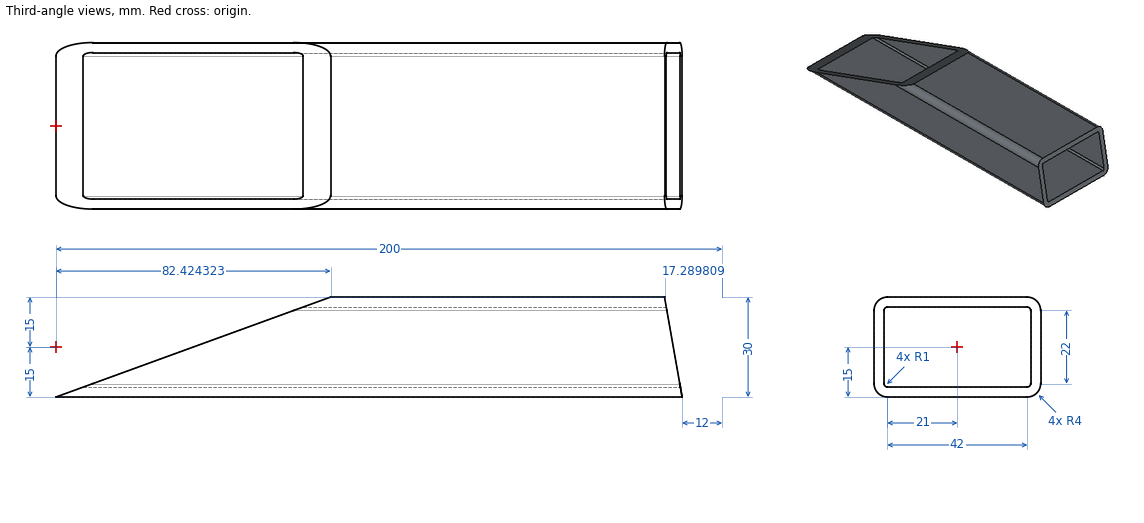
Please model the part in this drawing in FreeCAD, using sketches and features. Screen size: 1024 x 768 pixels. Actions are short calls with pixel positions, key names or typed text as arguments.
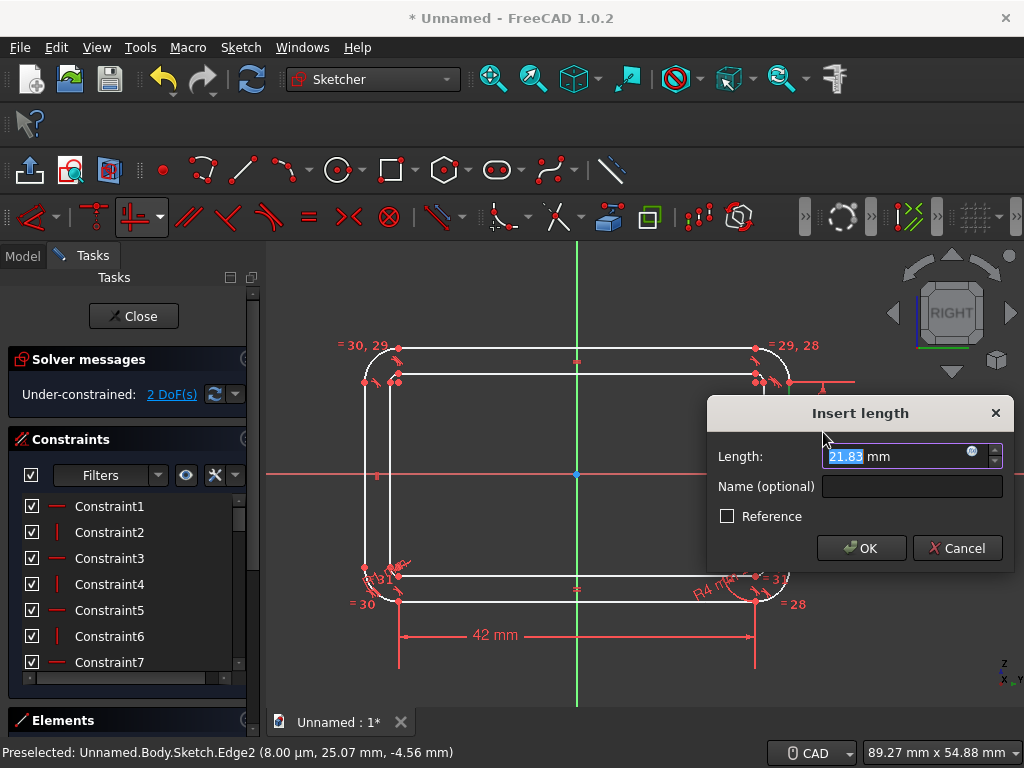
text(22)
key(Return)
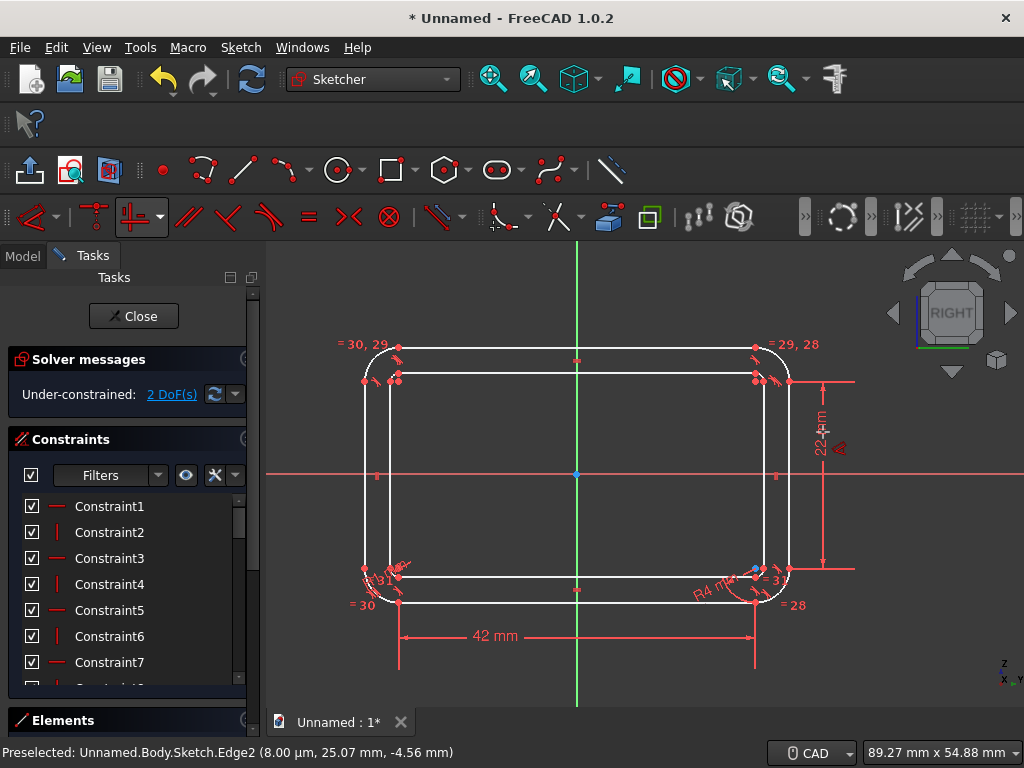
click(399, 603)
click(426, 637)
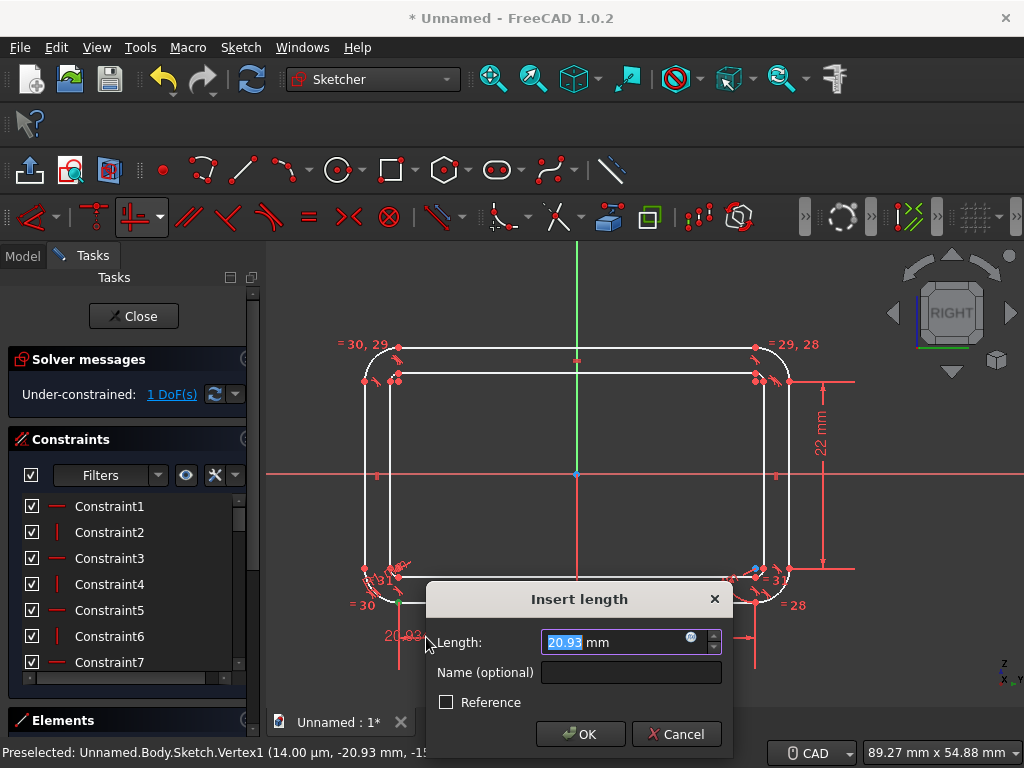
text(21)
key(Return)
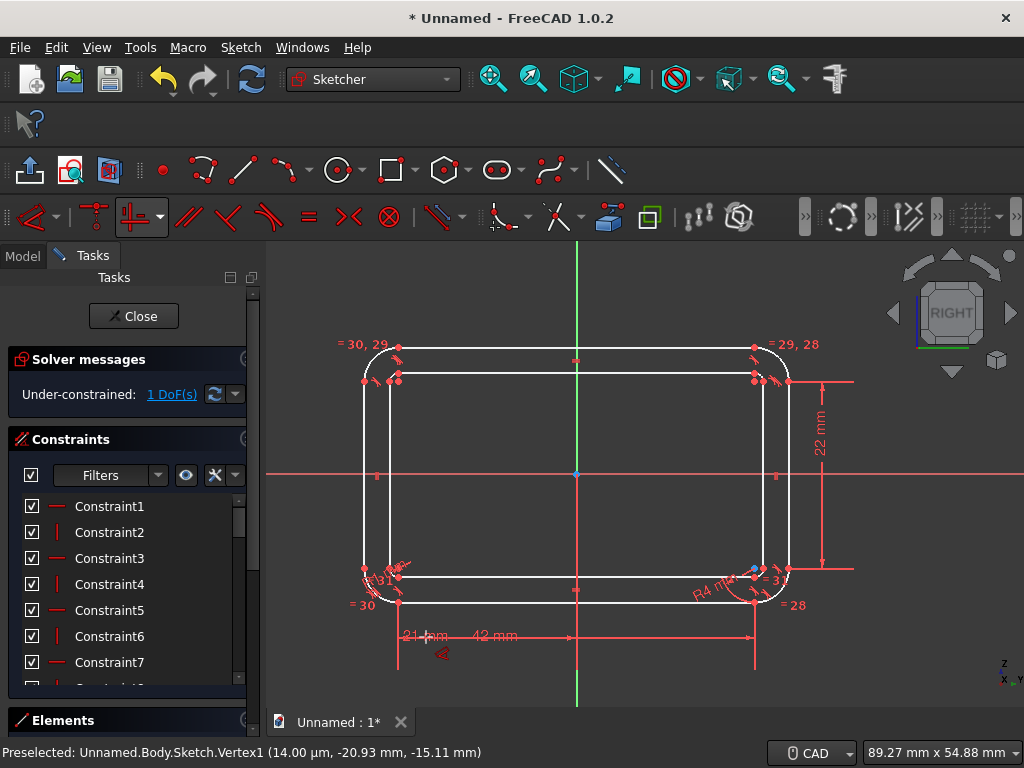
click(398, 603)
click(611, 538)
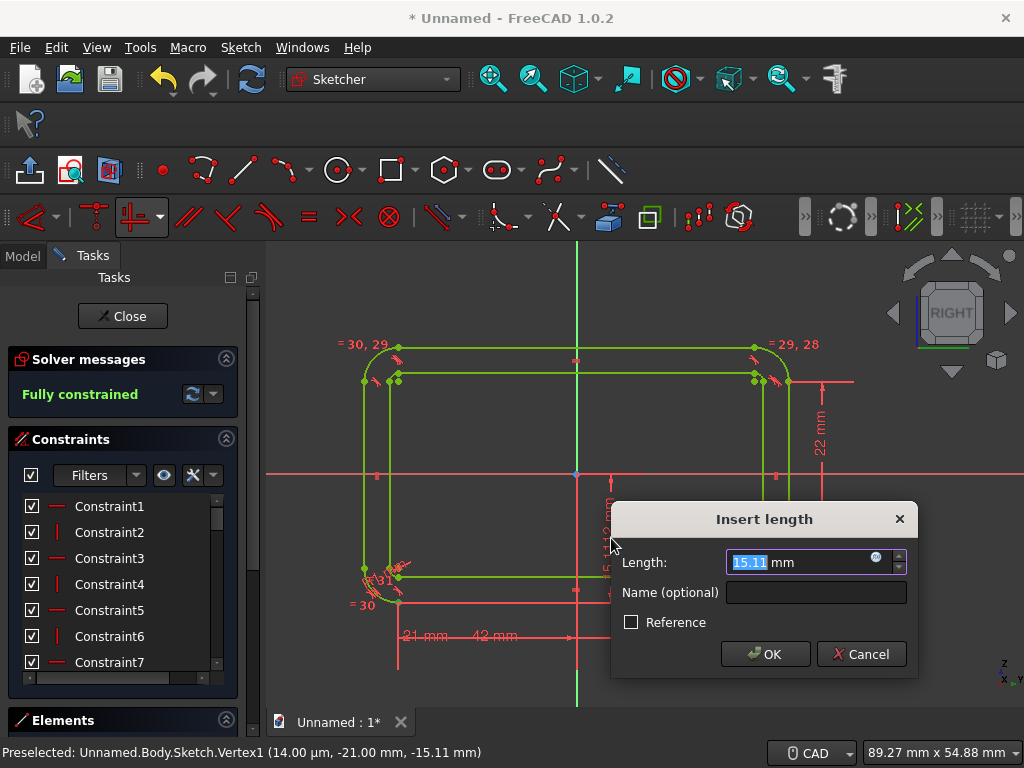
text(15)
key(Return)
key(Escape)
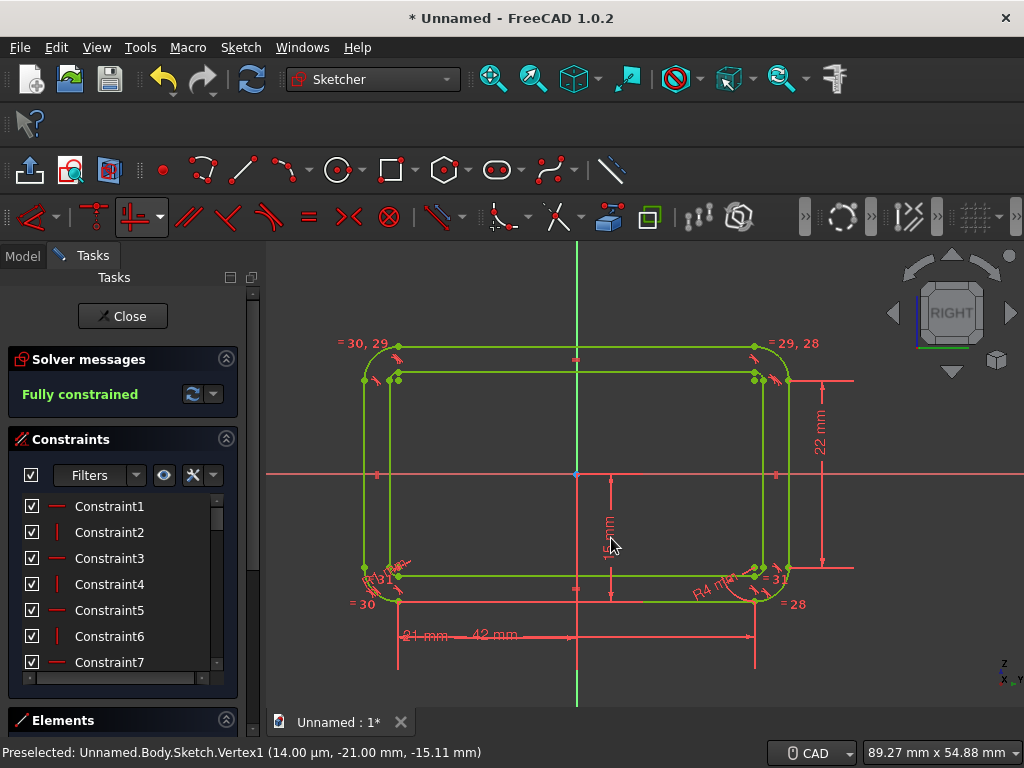
click(123, 316)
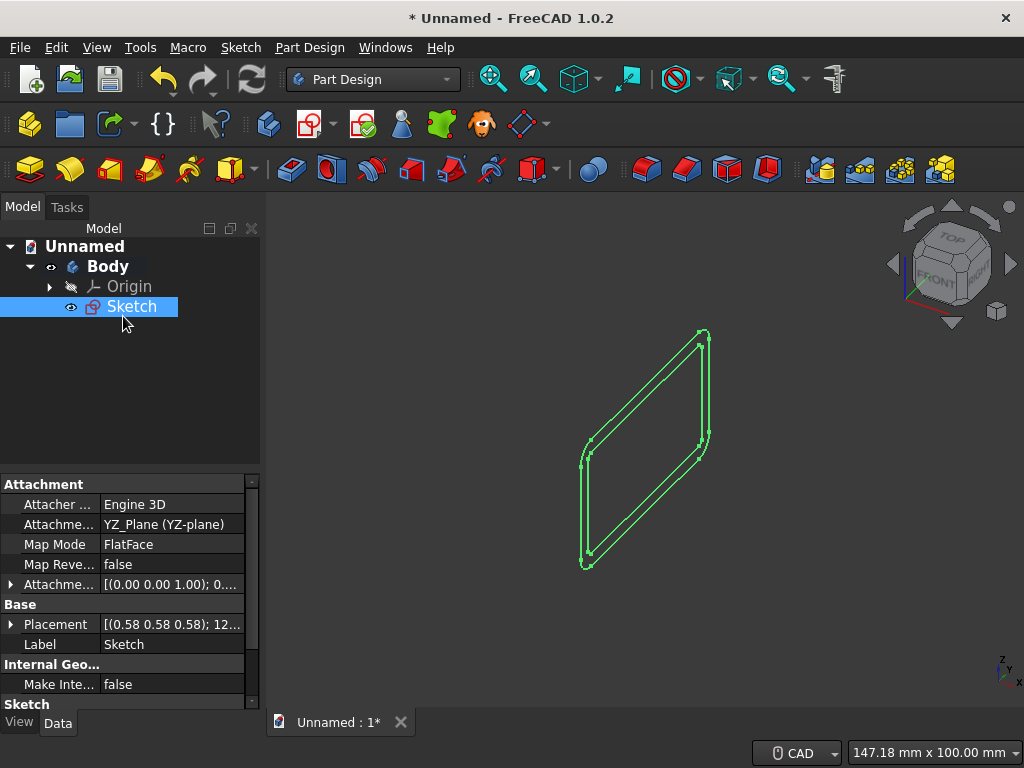
click(30, 170)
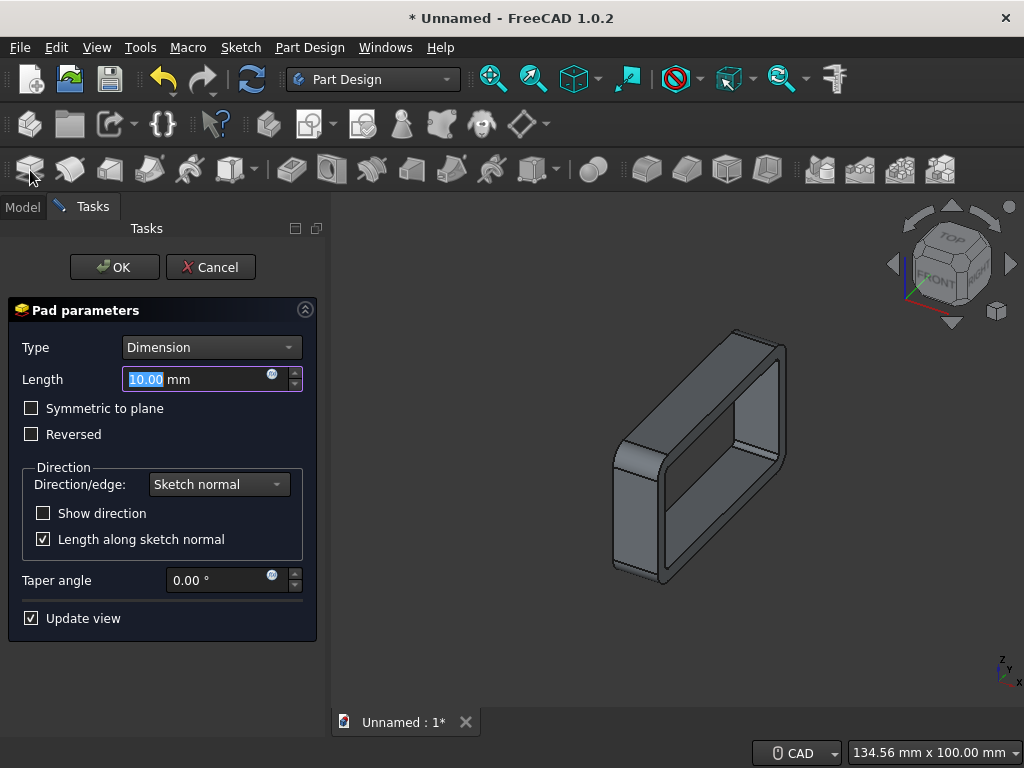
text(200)
key(Tab)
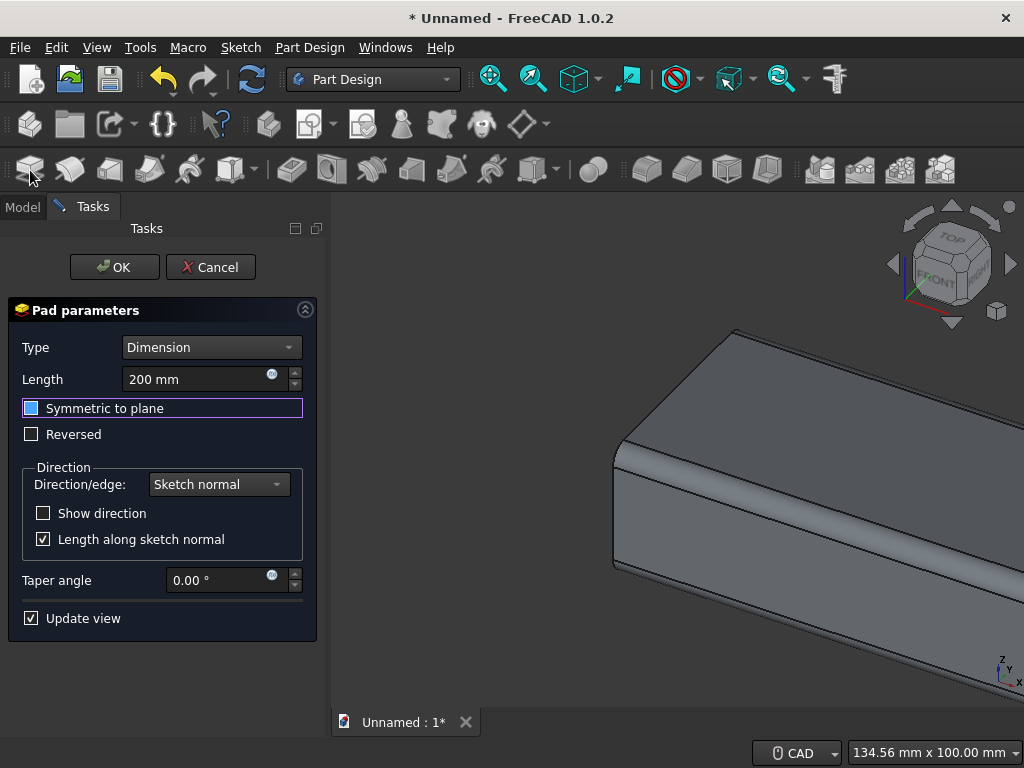
click(115, 267)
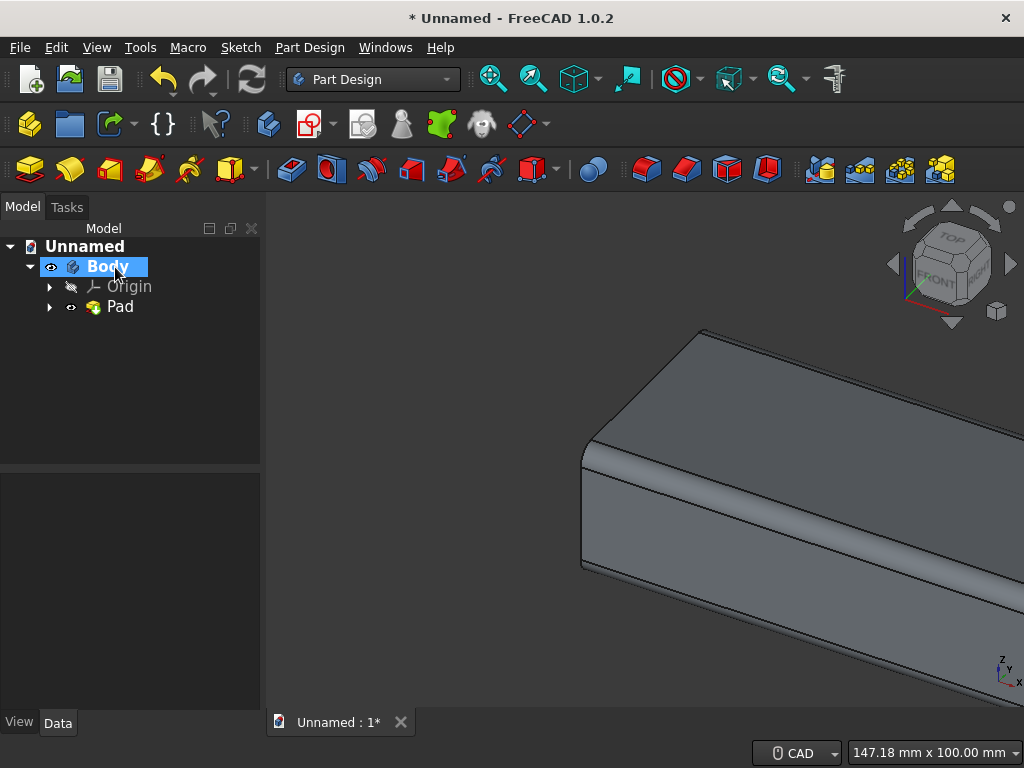
click(494, 80)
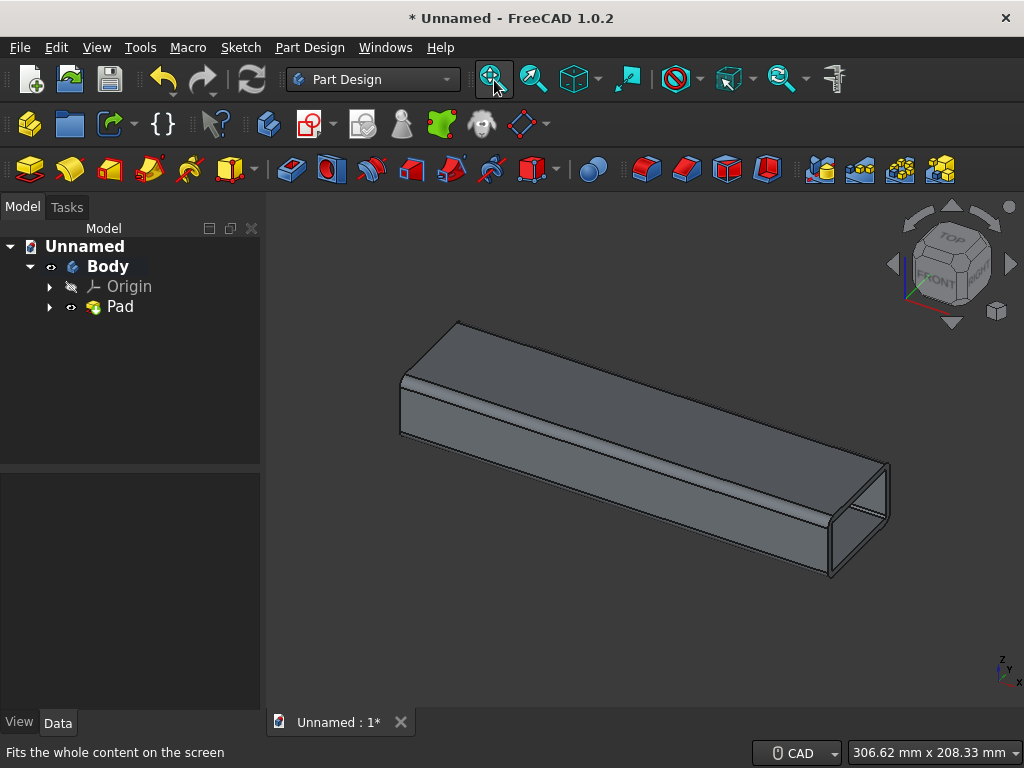
key(4)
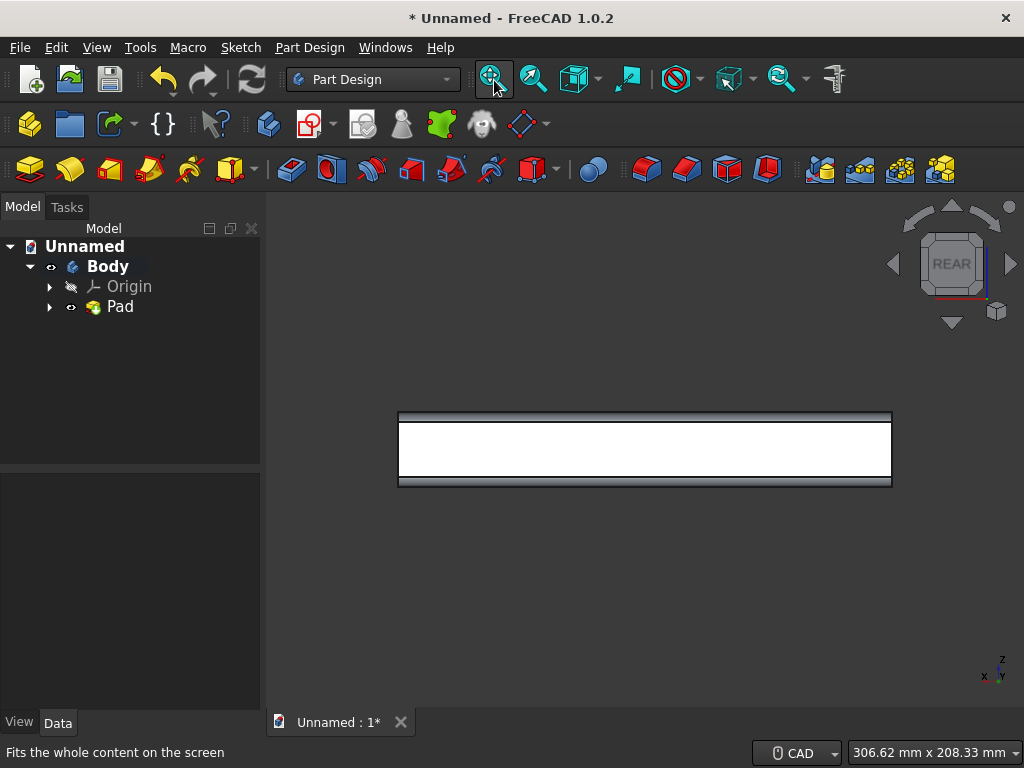
click(645, 449)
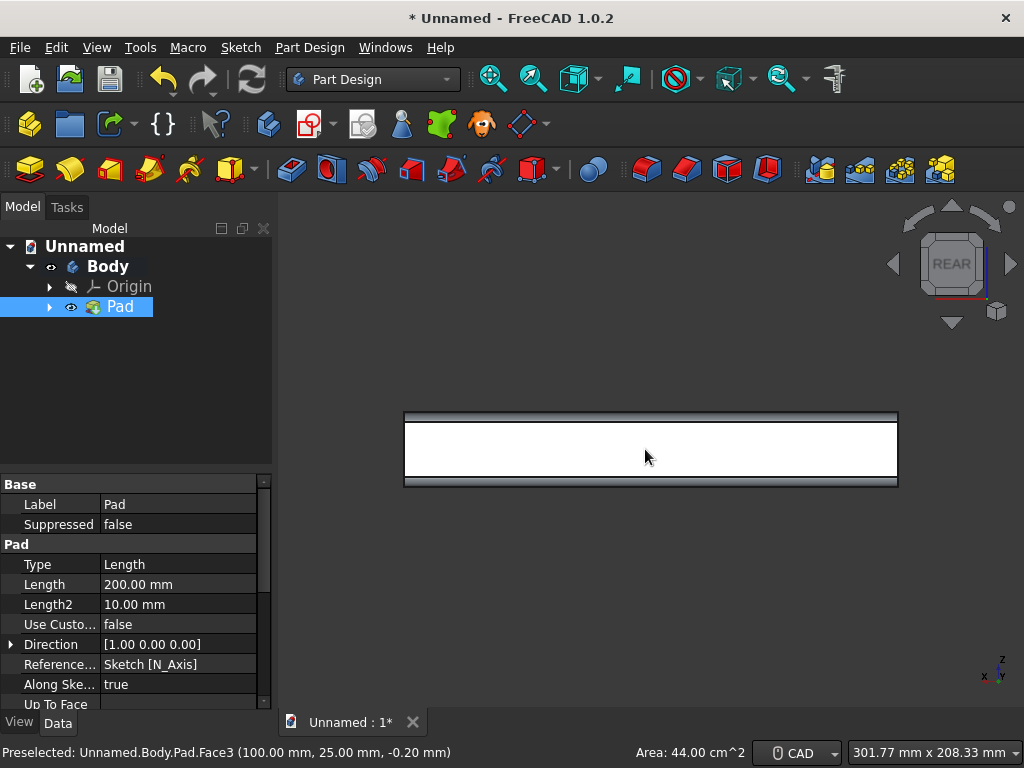
click(310, 124)